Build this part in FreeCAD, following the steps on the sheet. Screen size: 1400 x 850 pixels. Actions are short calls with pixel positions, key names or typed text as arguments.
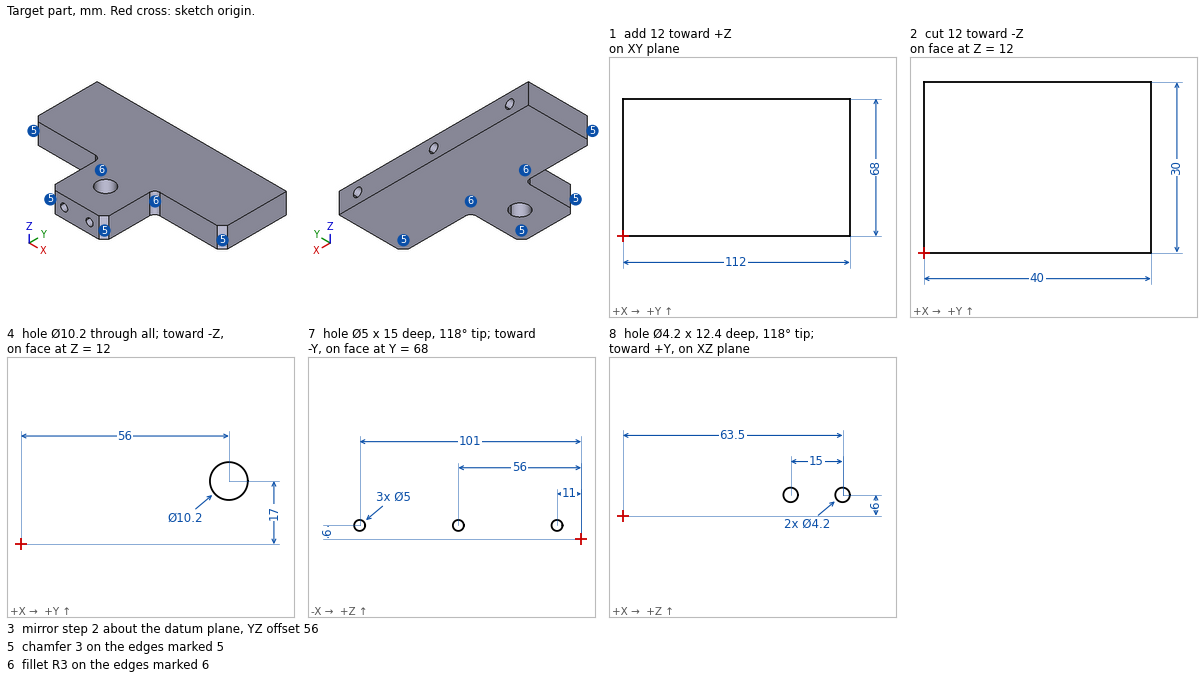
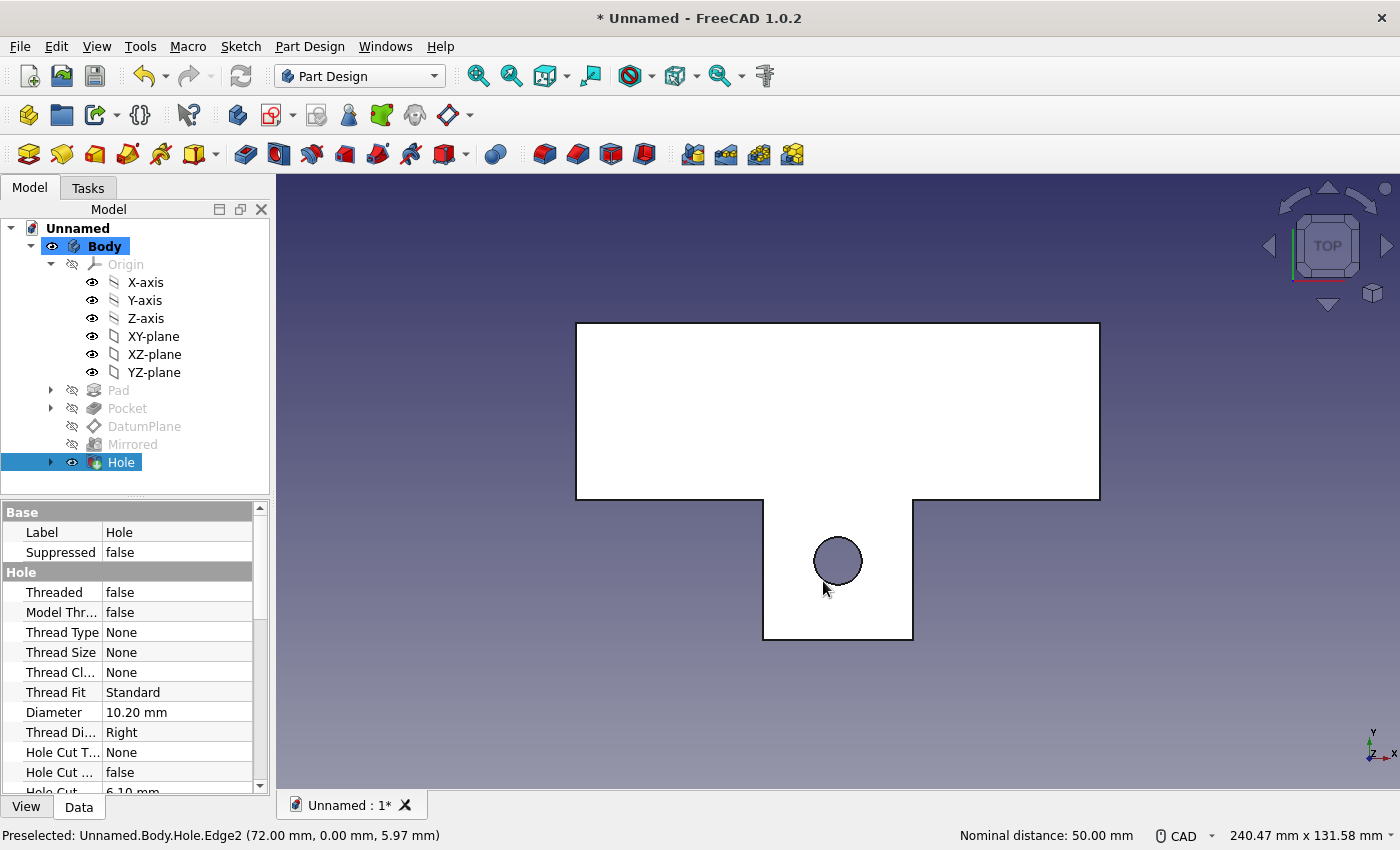
key(1)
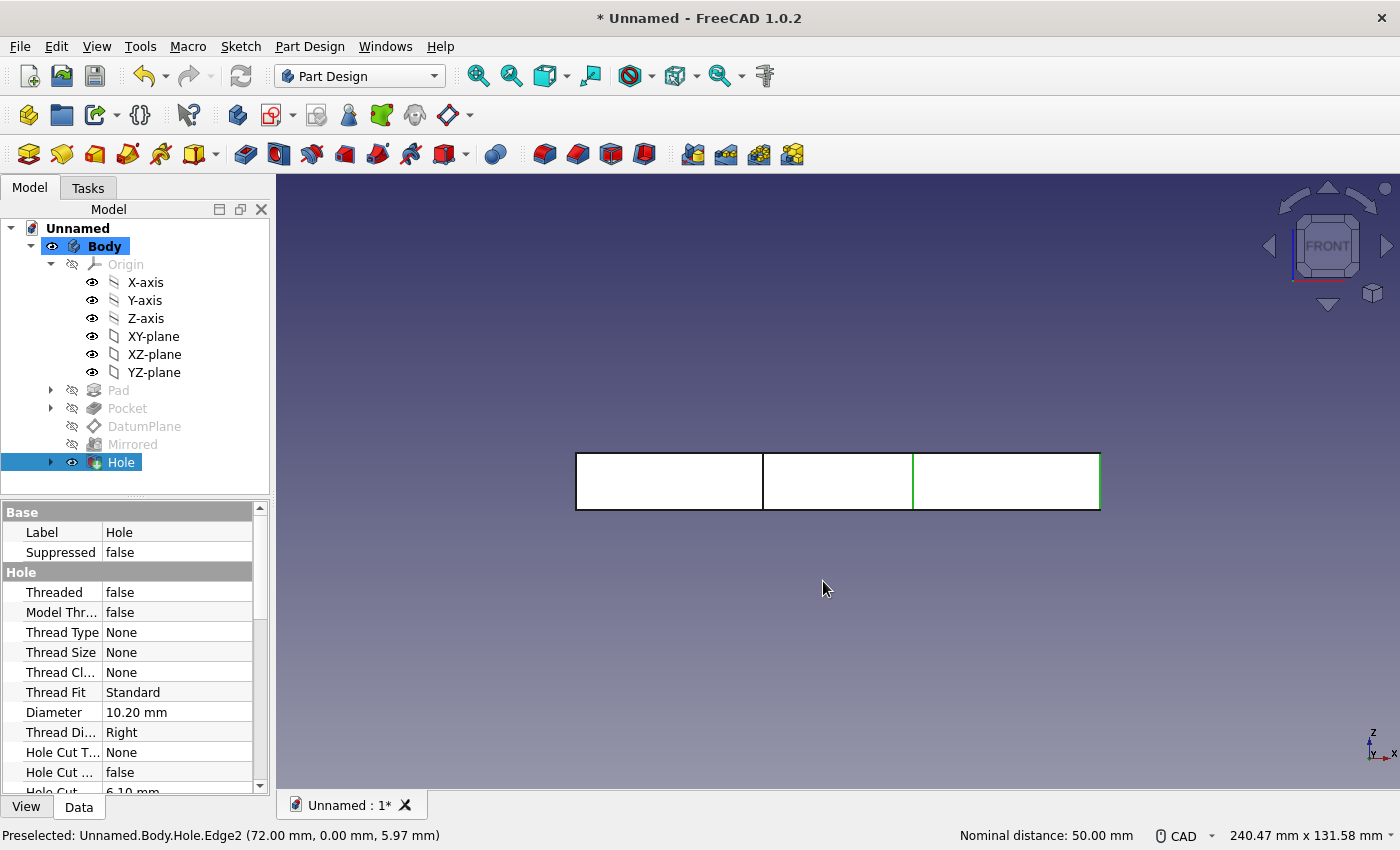
click(576, 480, ctrl)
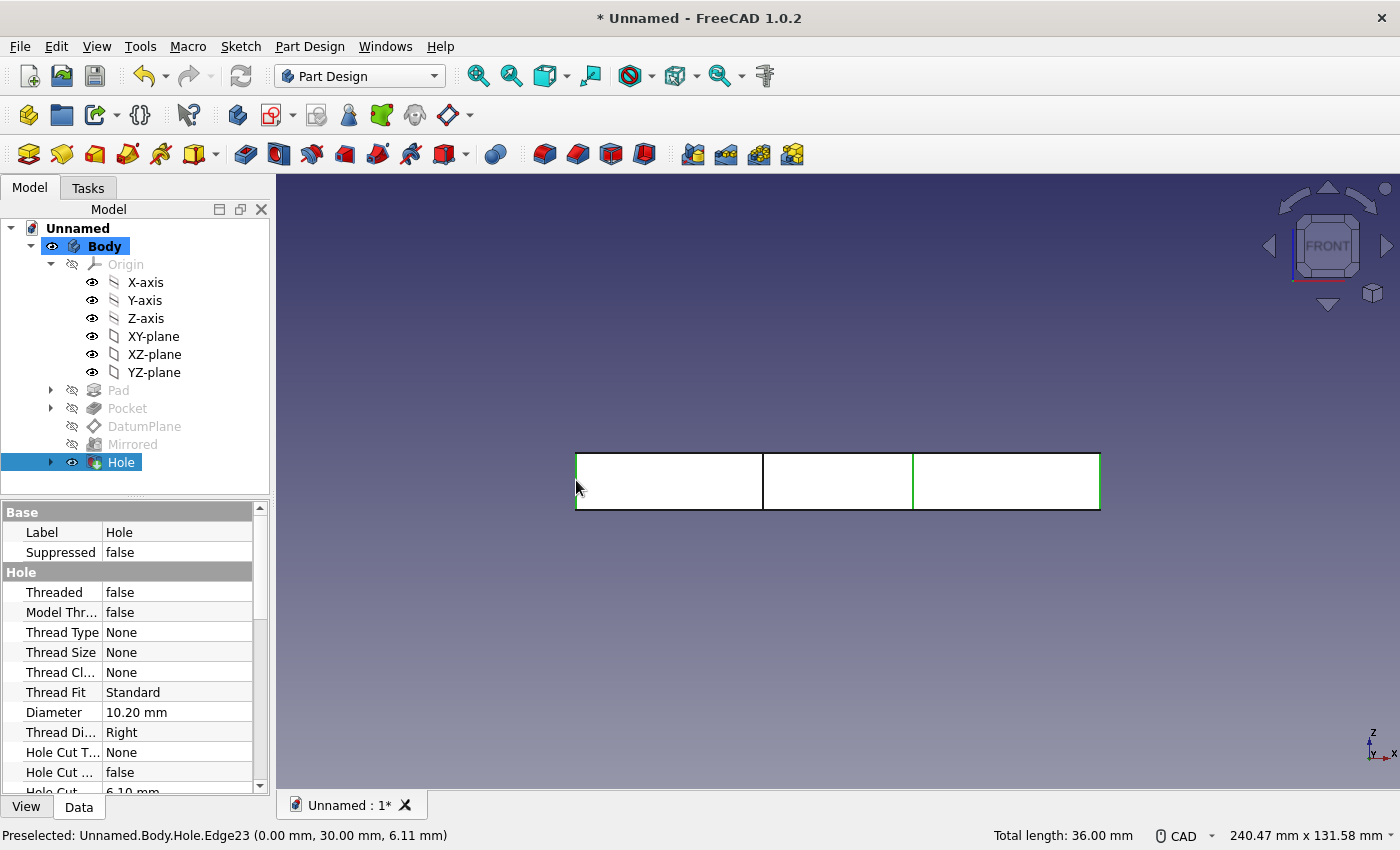
click(763, 480, ctrl)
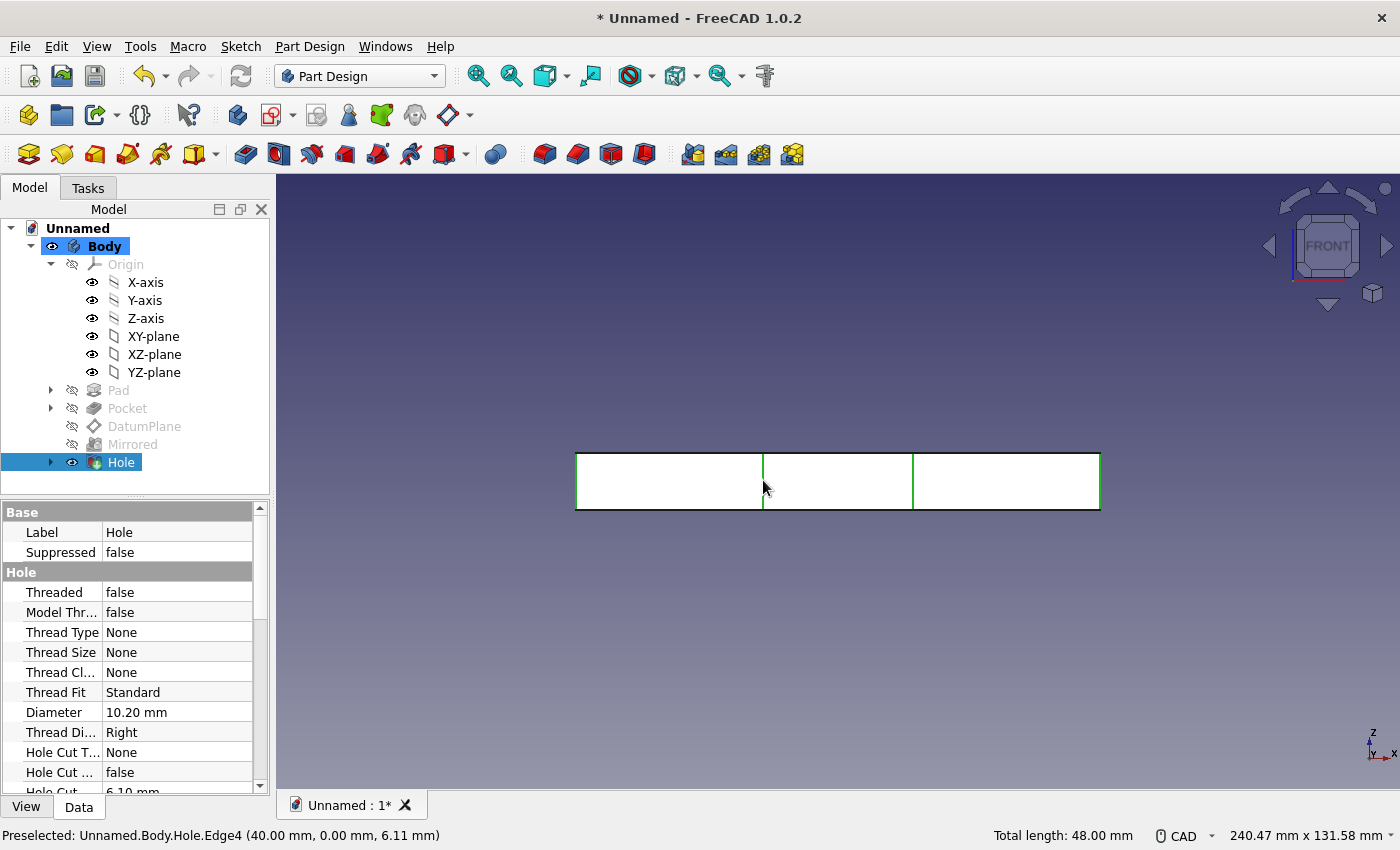
click(578, 154)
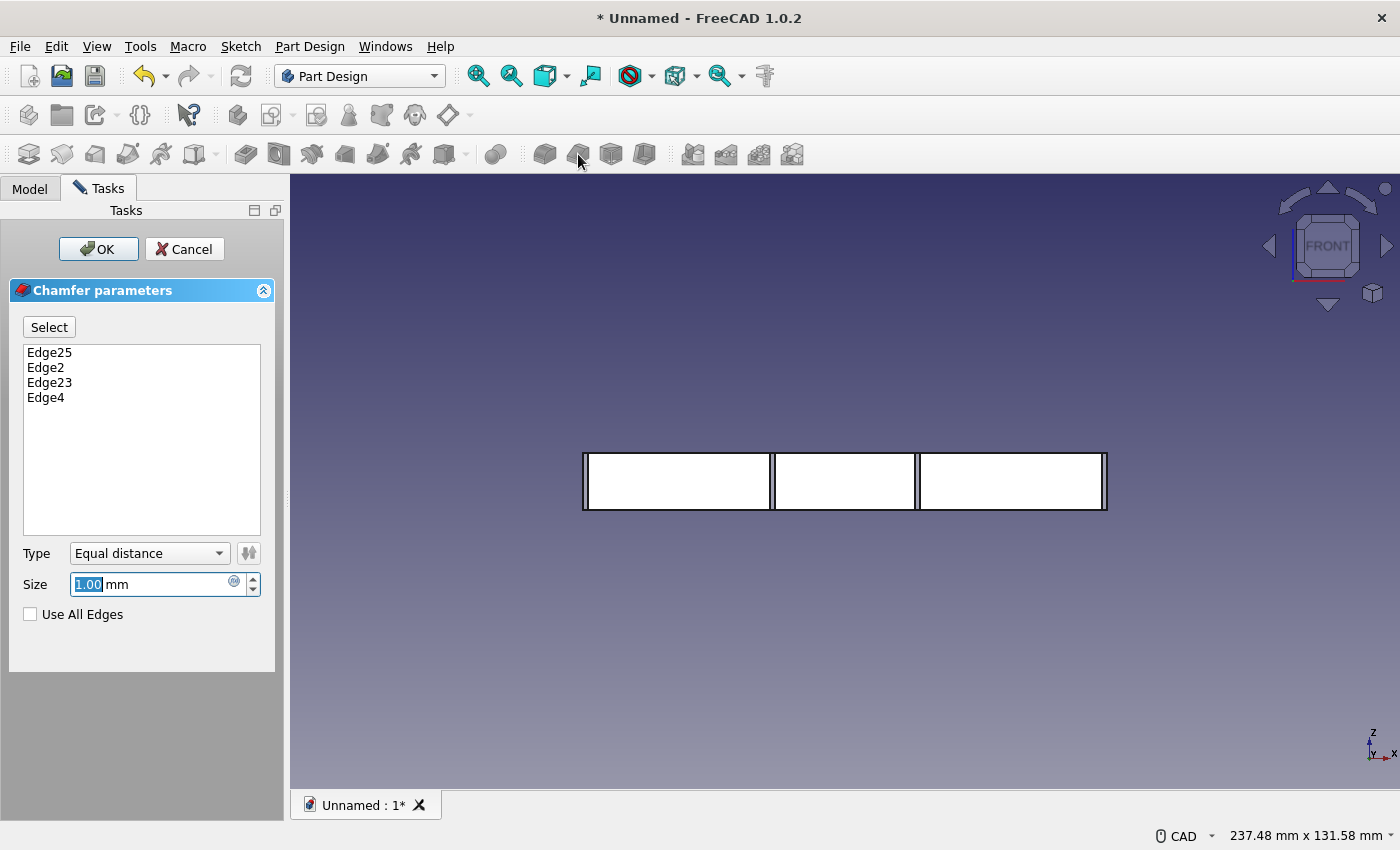
text(3)
key(Tab)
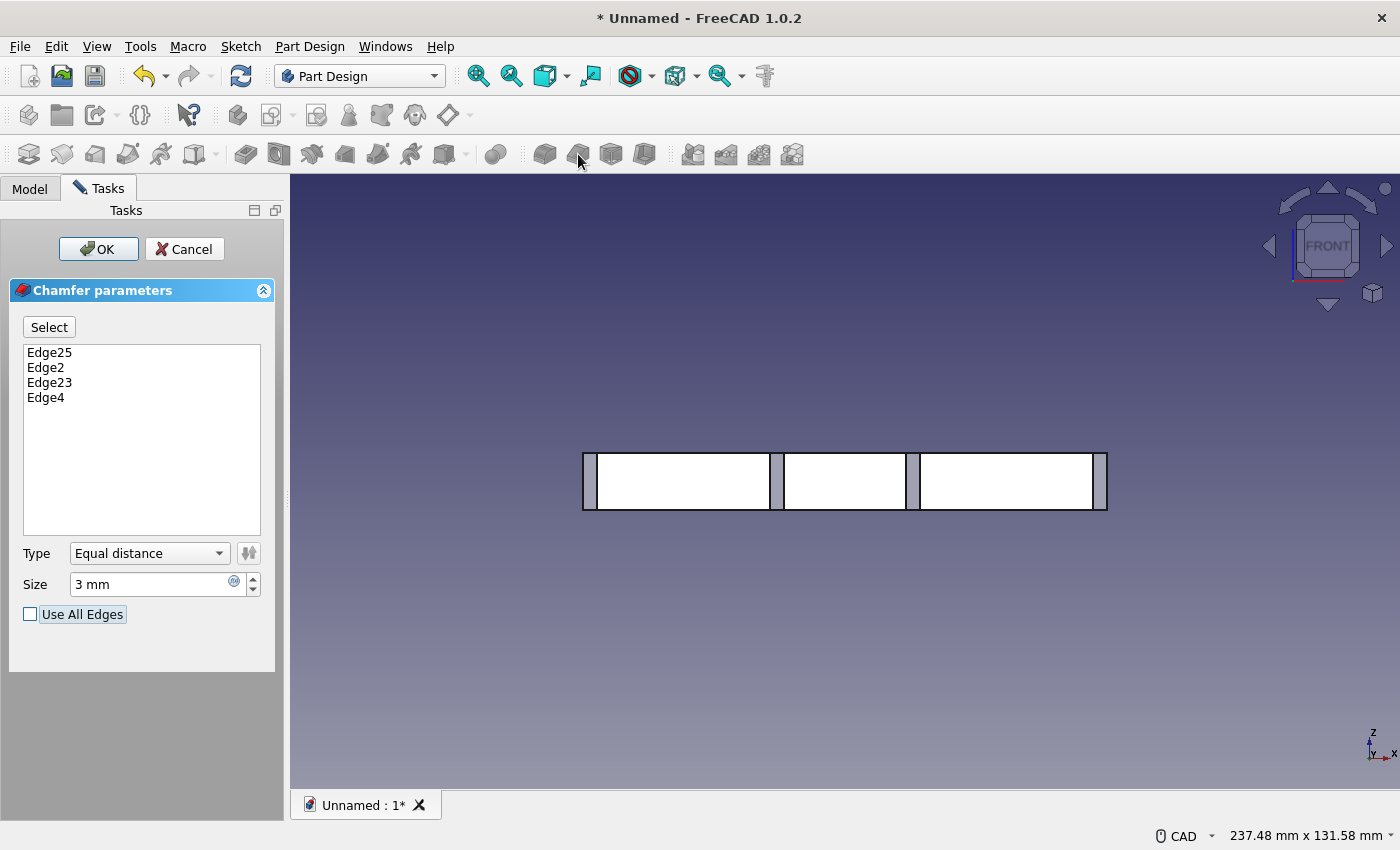
click(99, 249)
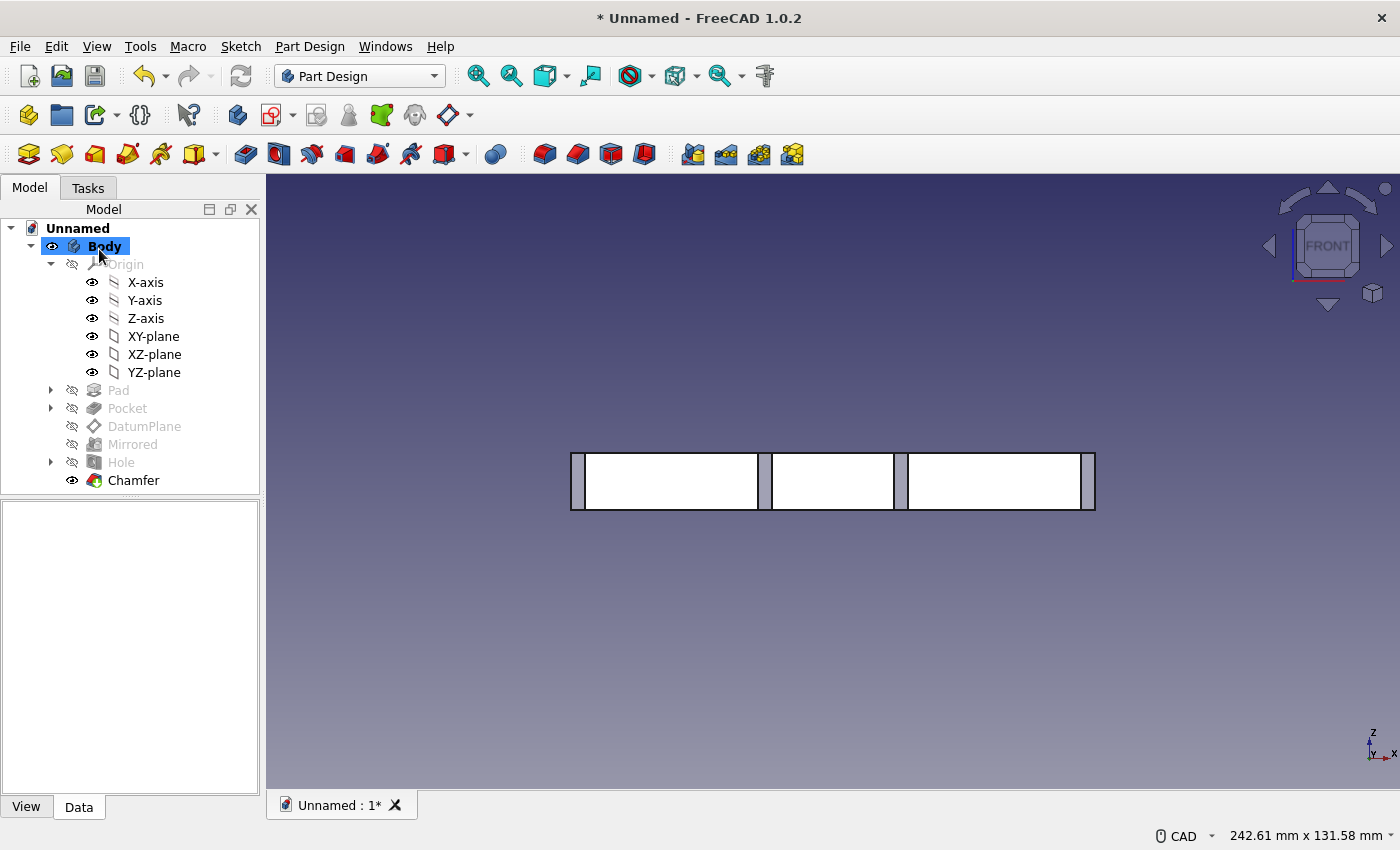
key(0)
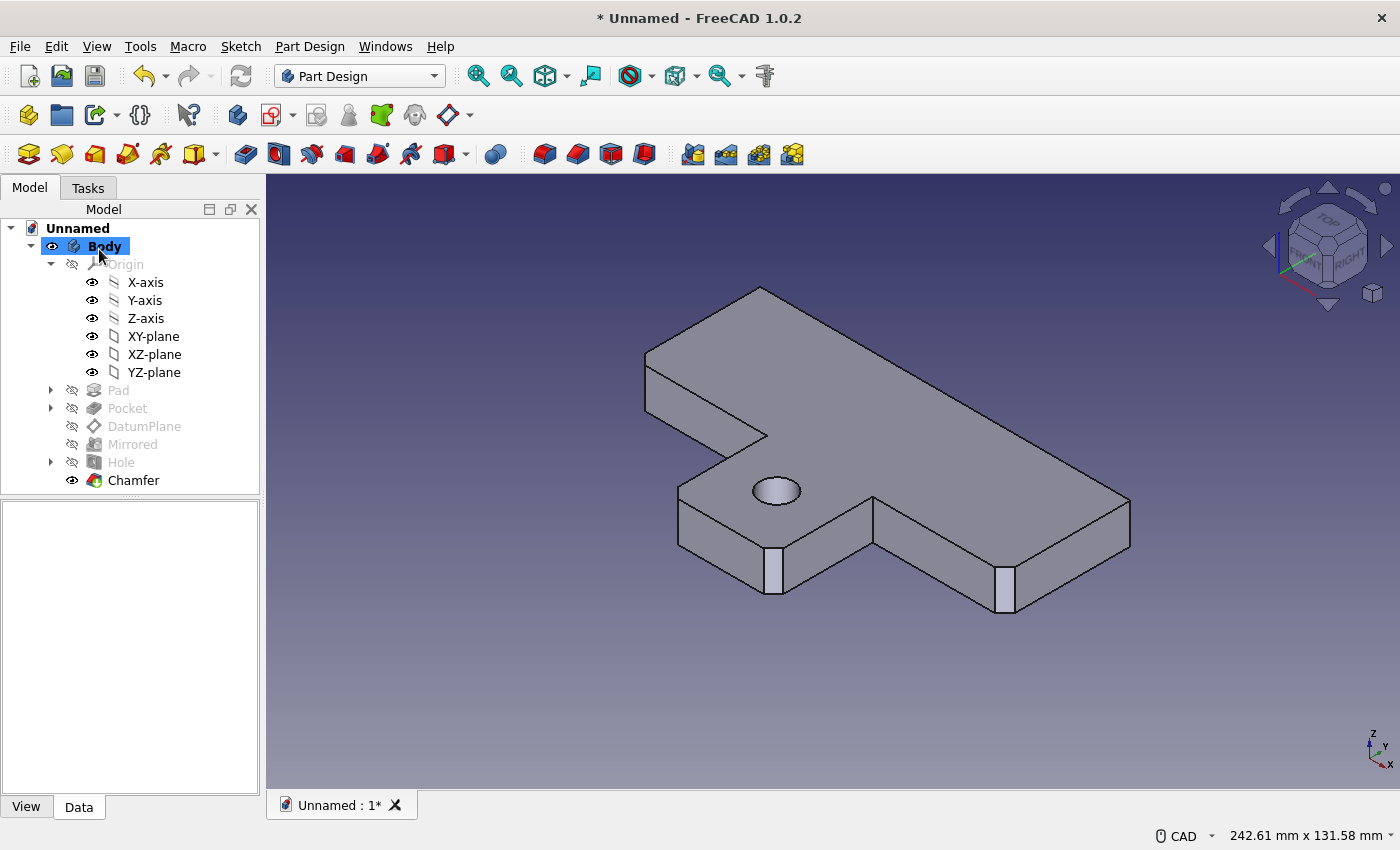
key(2)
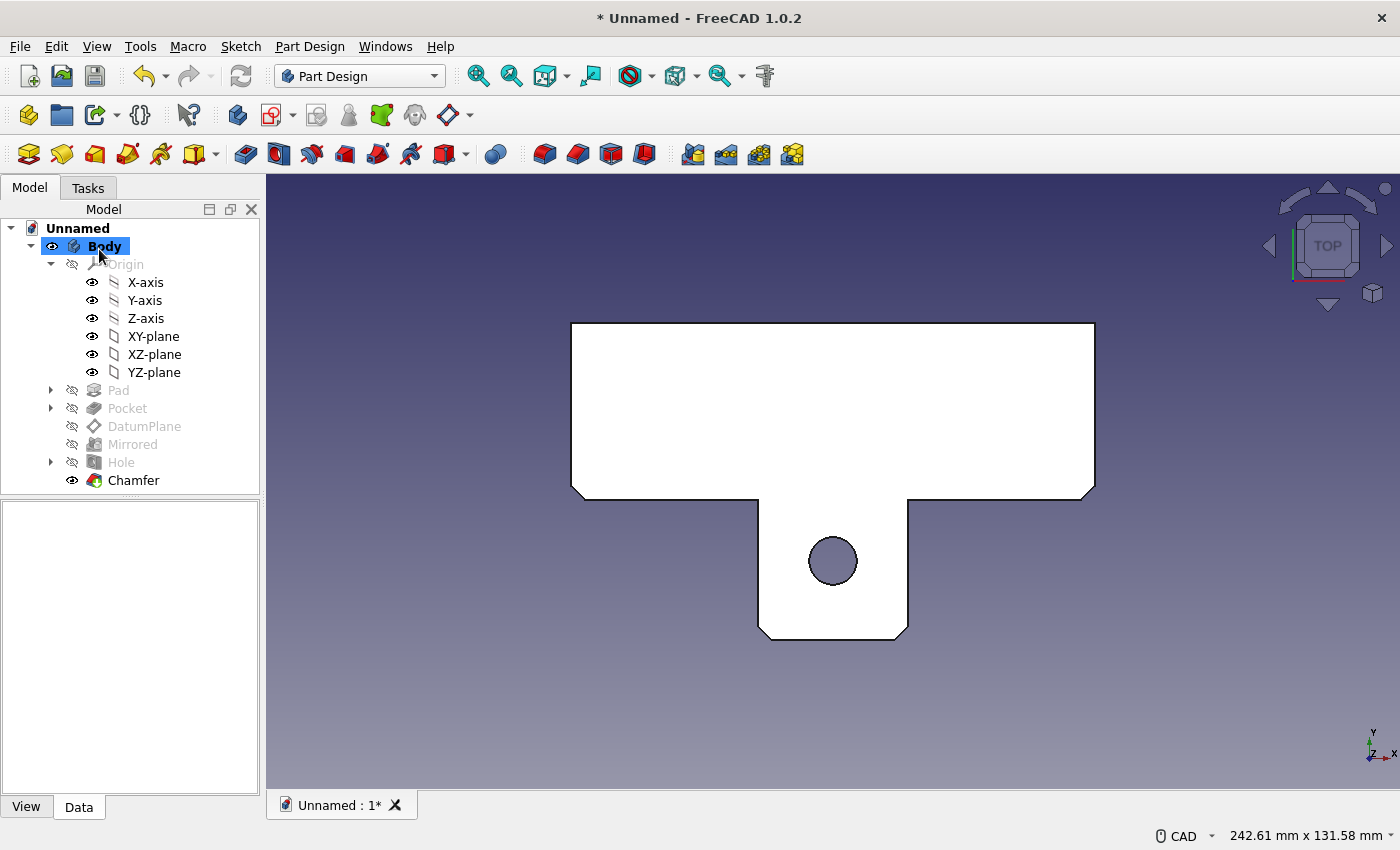
key(1)